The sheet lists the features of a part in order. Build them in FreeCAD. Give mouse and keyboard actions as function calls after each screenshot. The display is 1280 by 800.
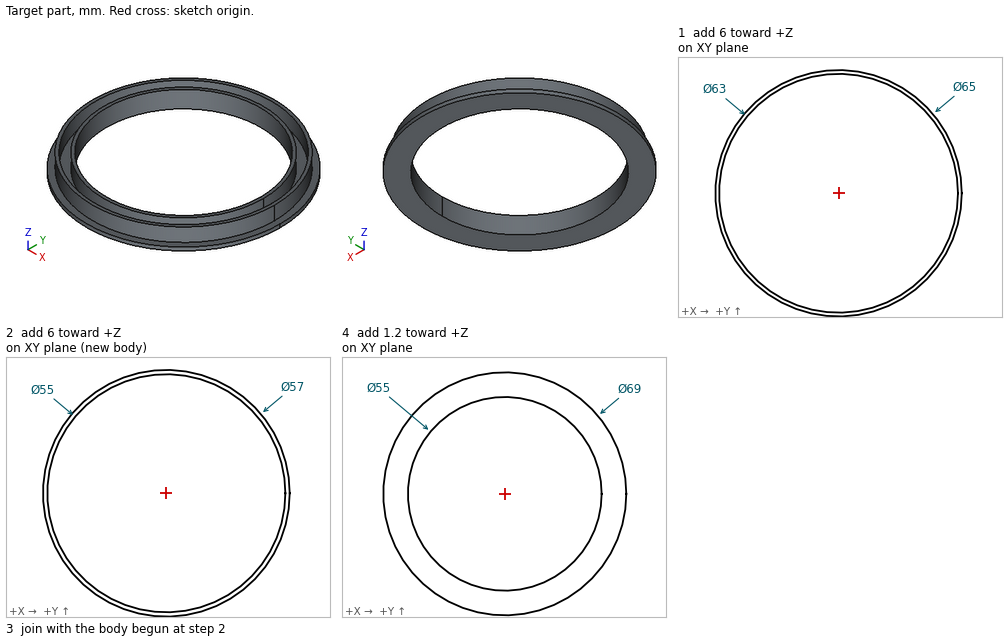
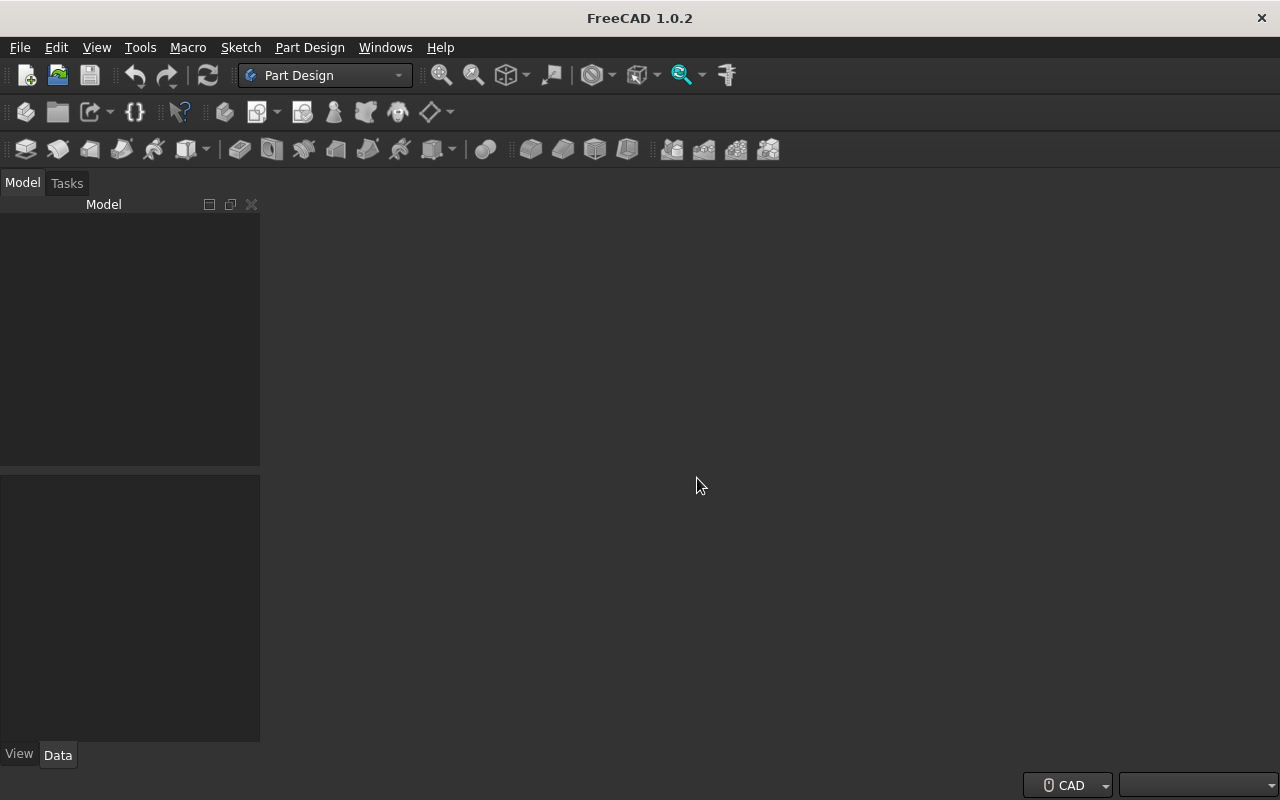
click(26, 76)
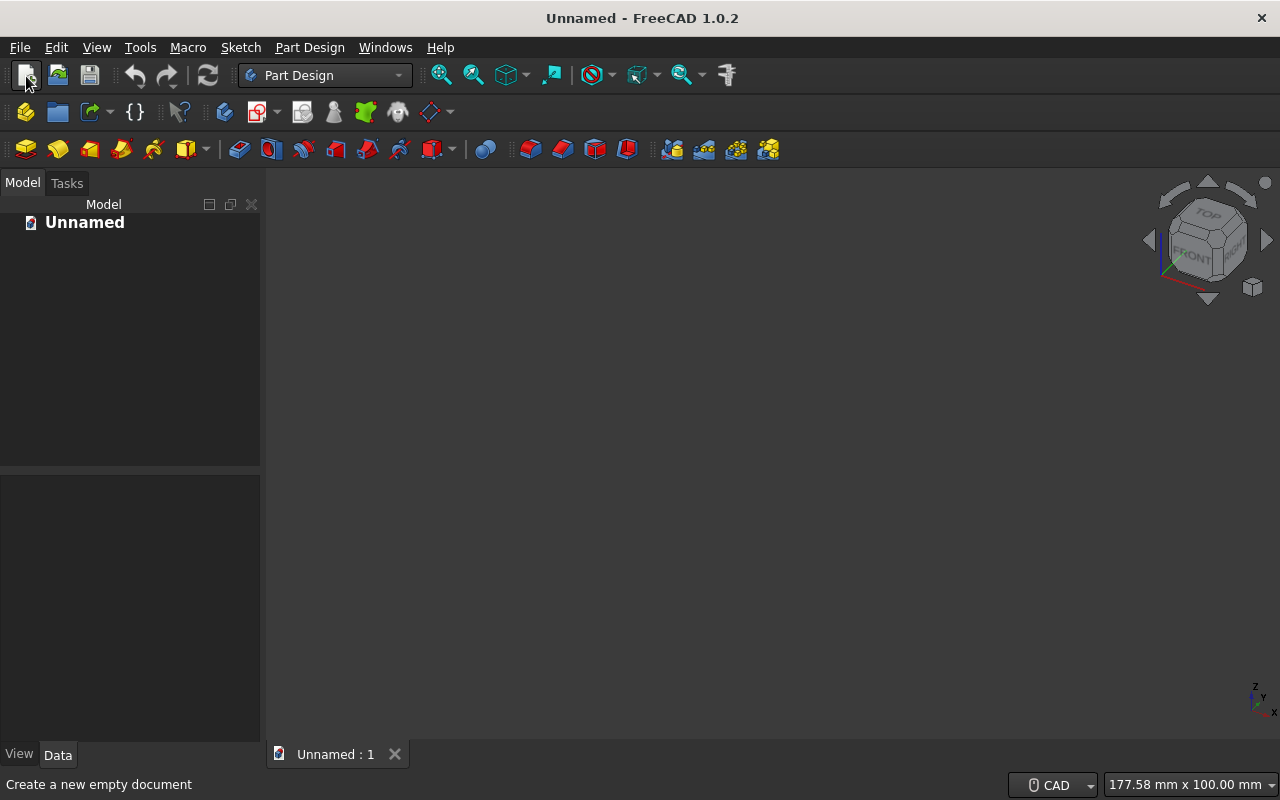
click(258, 112)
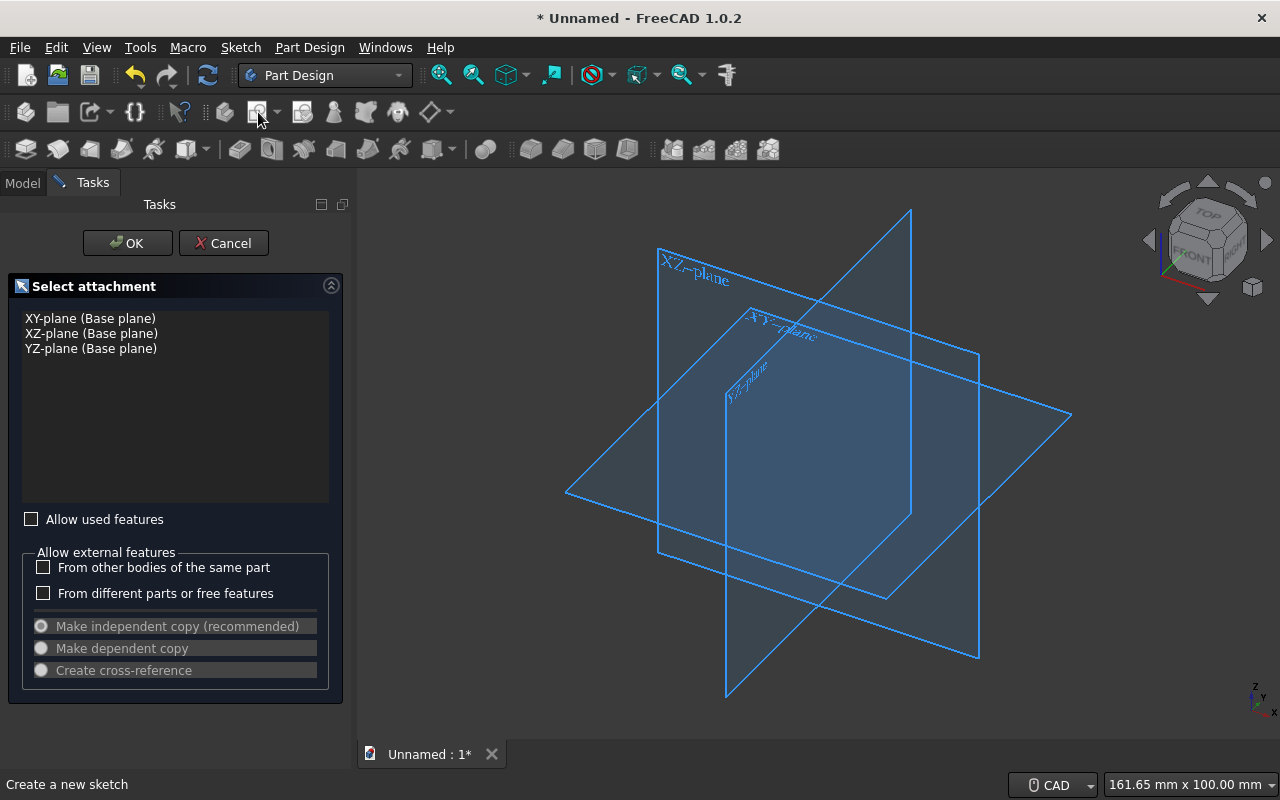
click(82, 318)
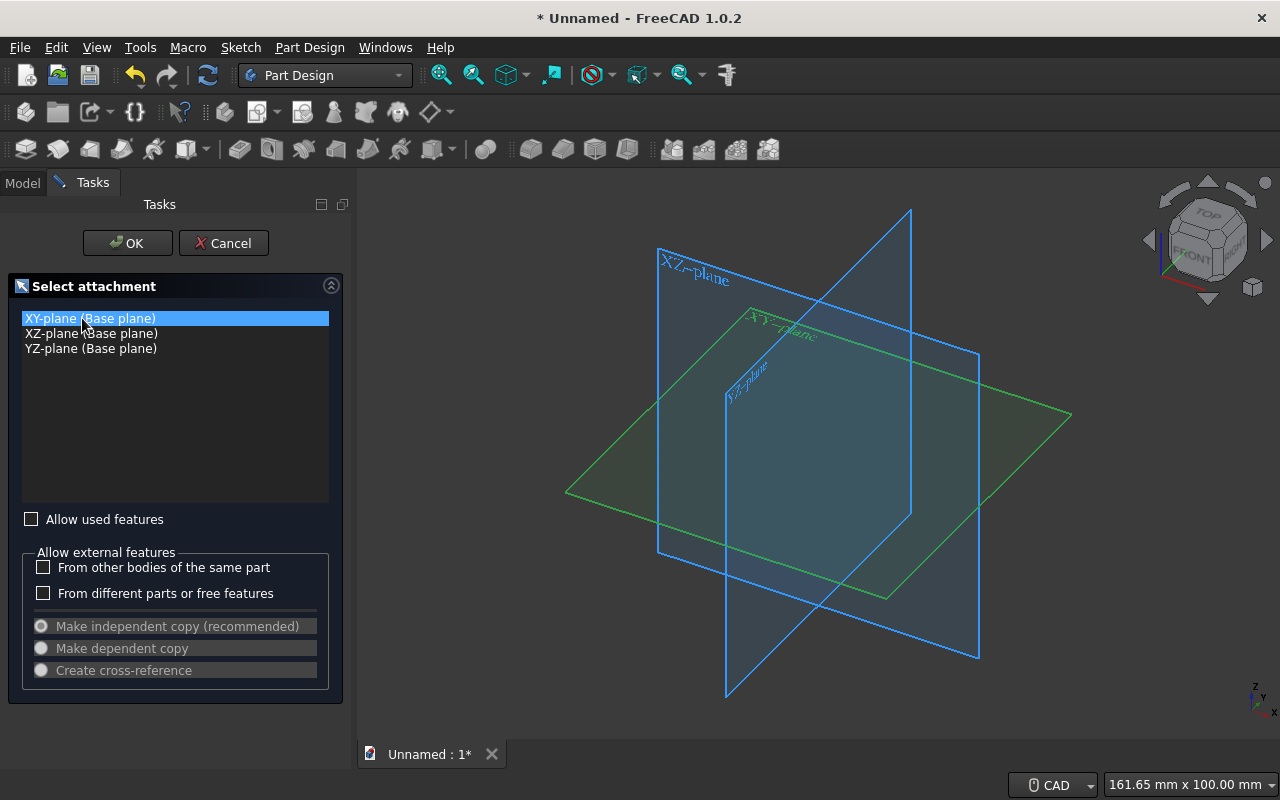
click(128, 243)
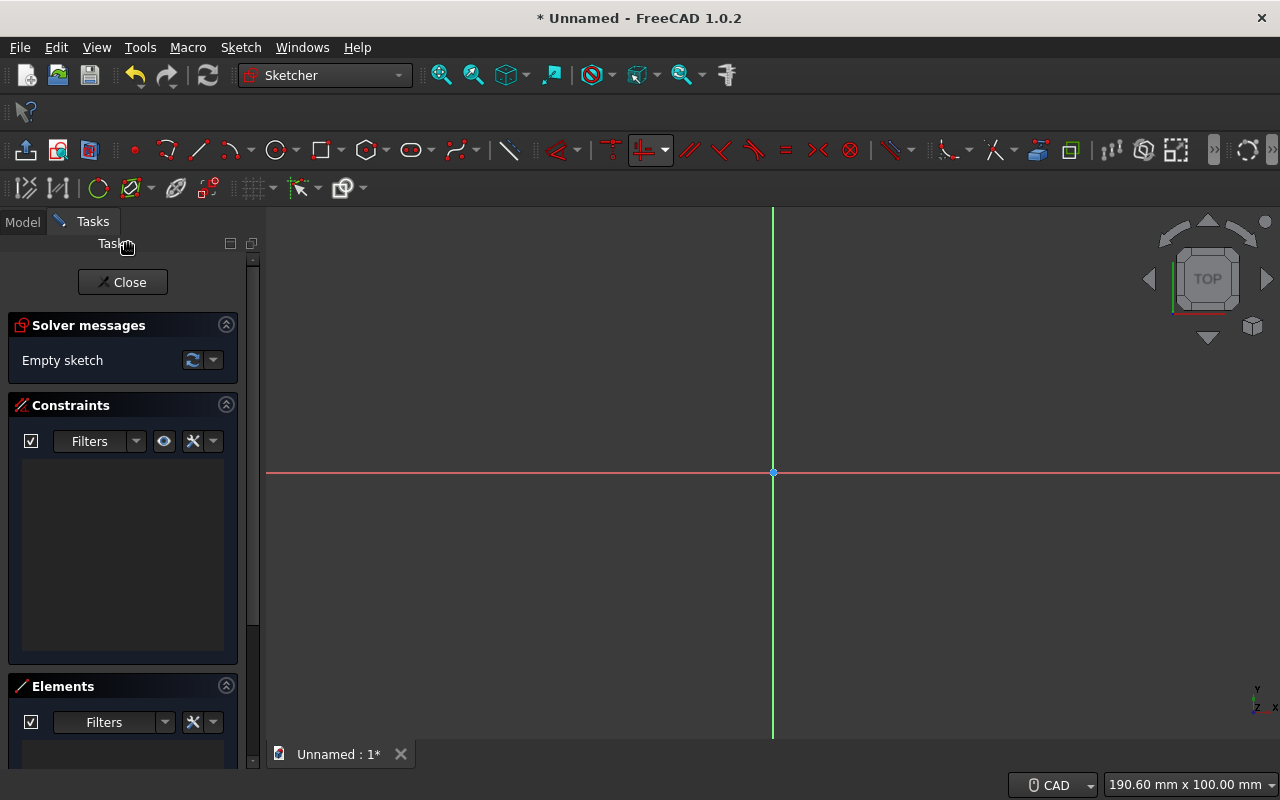
click(276, 150)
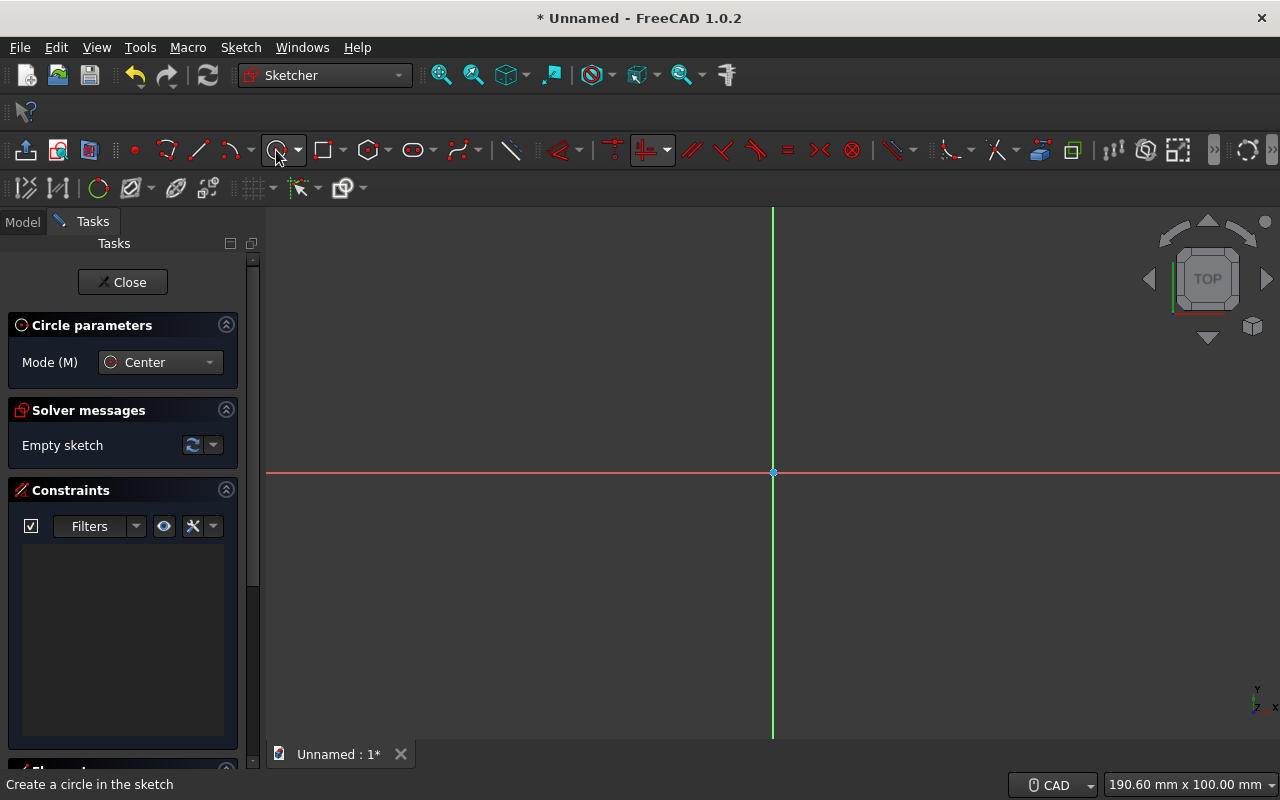
click(773, 473)
move(895, 351)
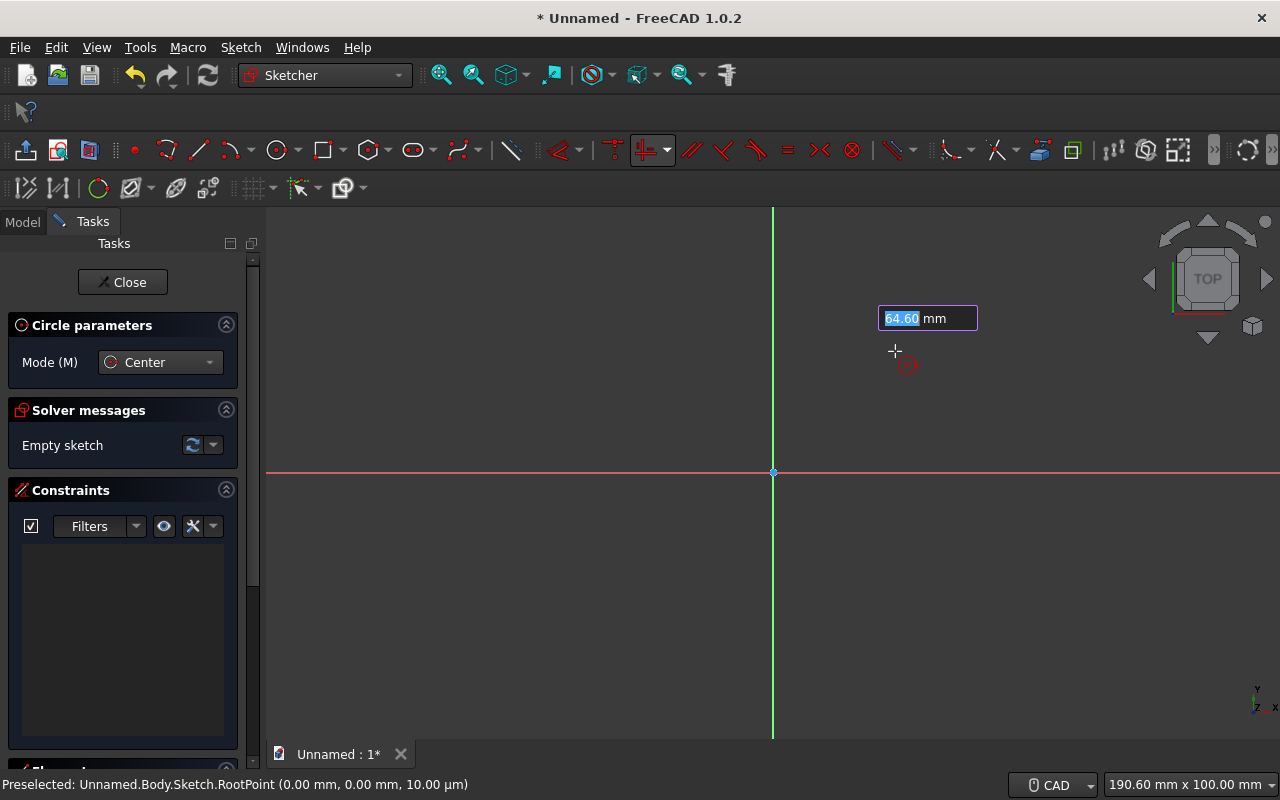
text(65)
key(Return)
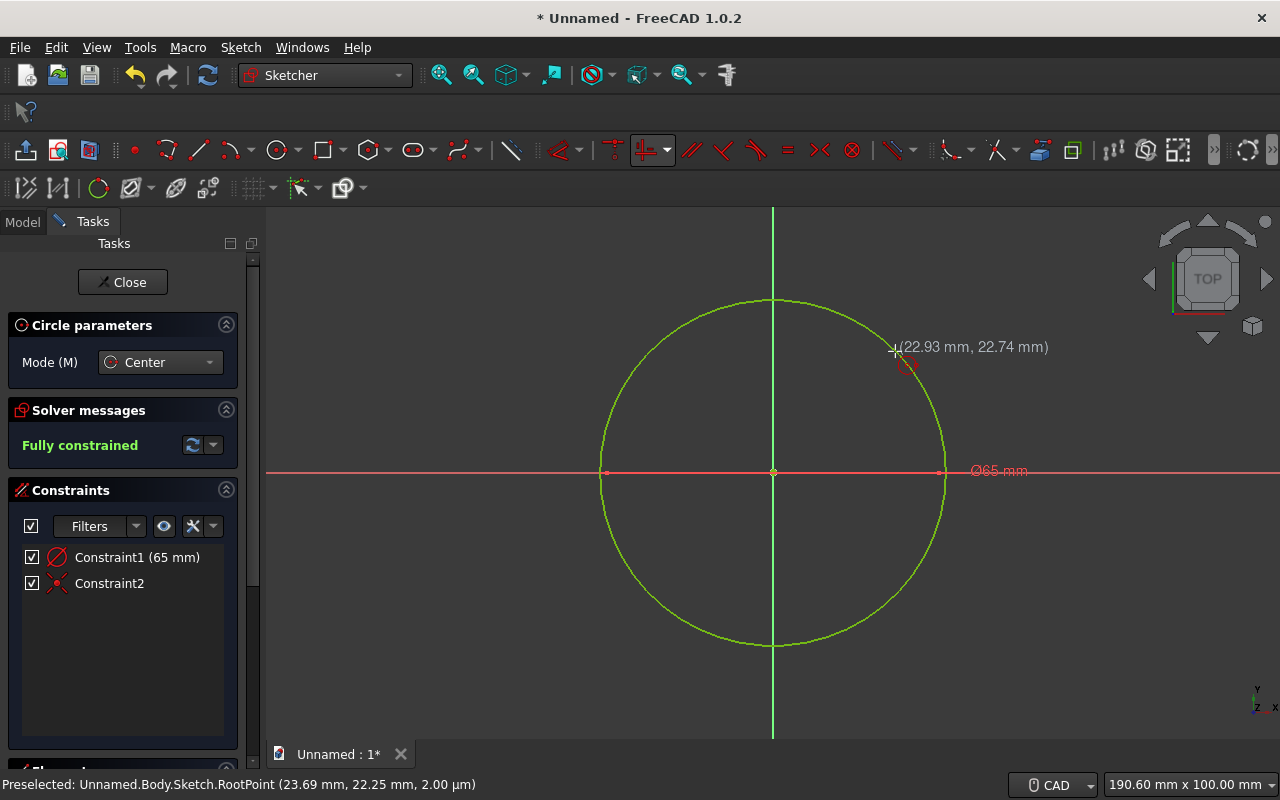
click(773, 473)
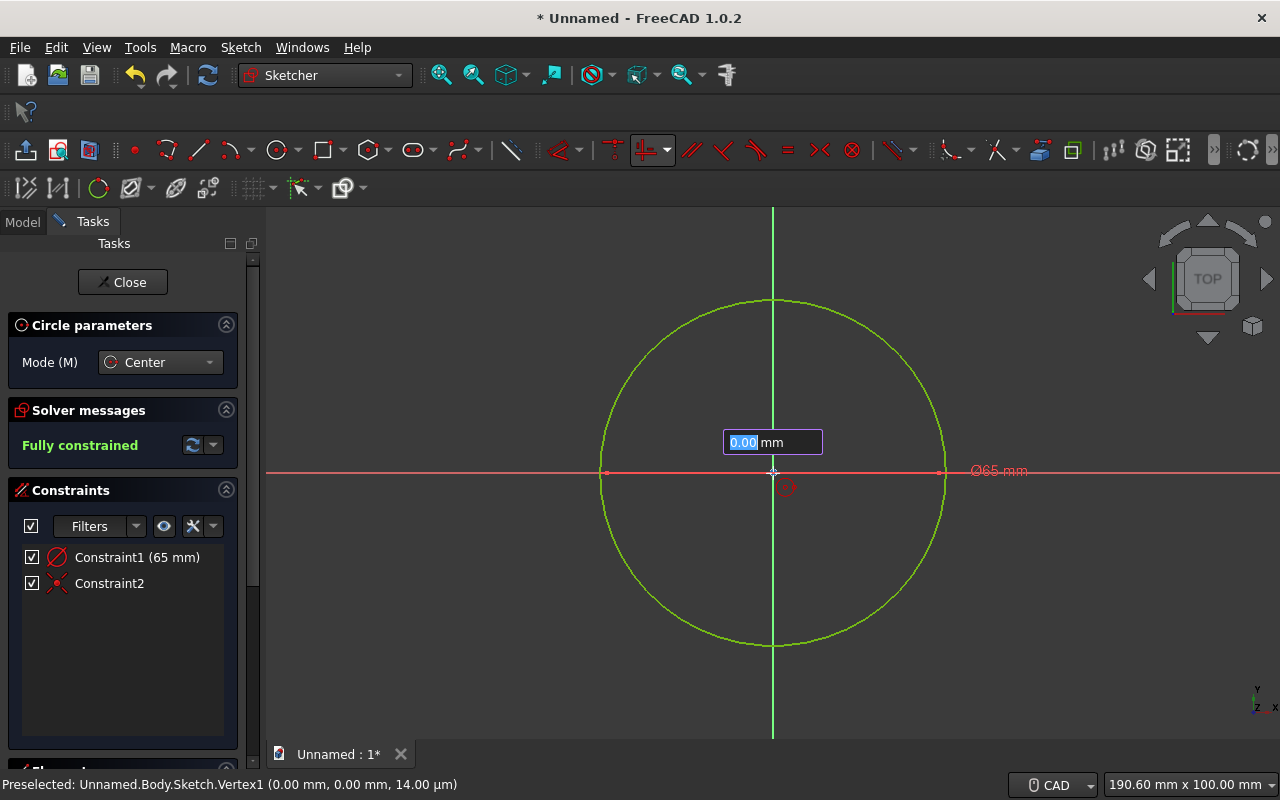
scroll(891, 355, up, 6)
move(891, 353)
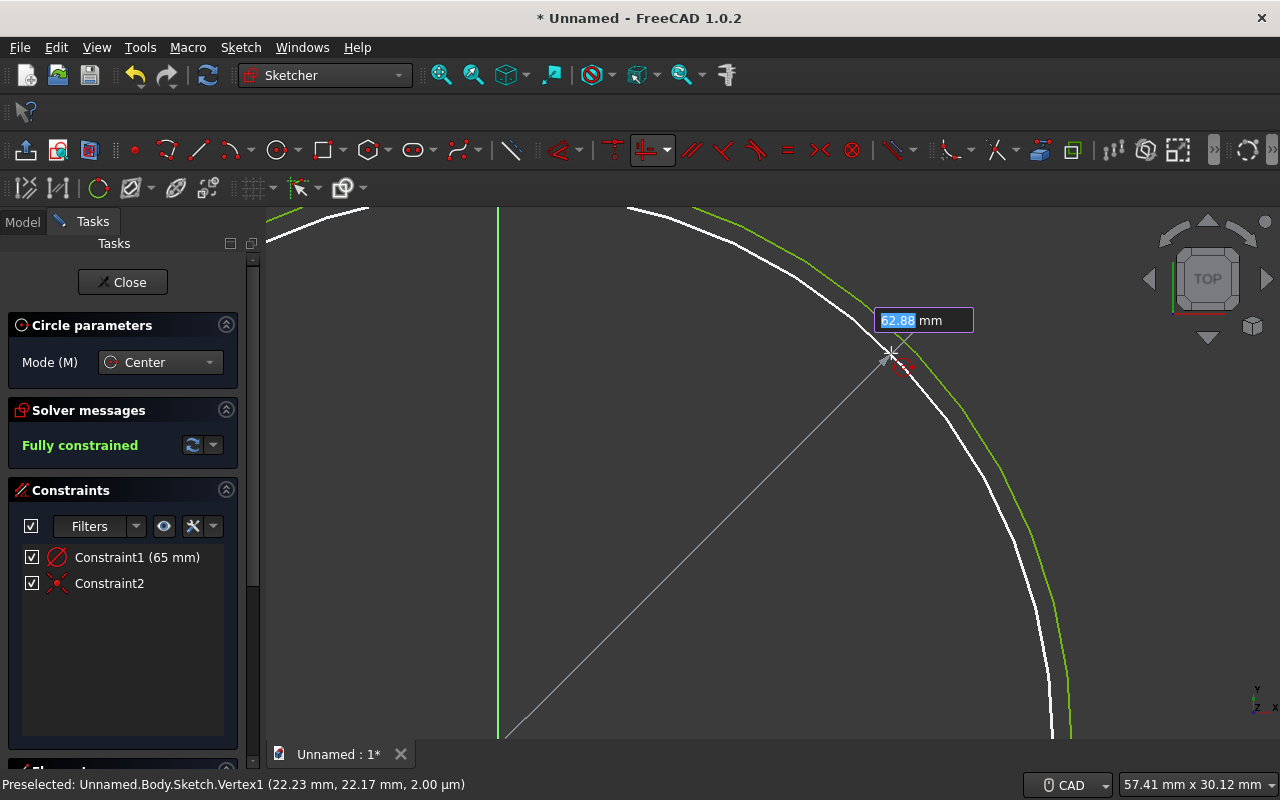
text(63)
key(Return)
key(Escape)